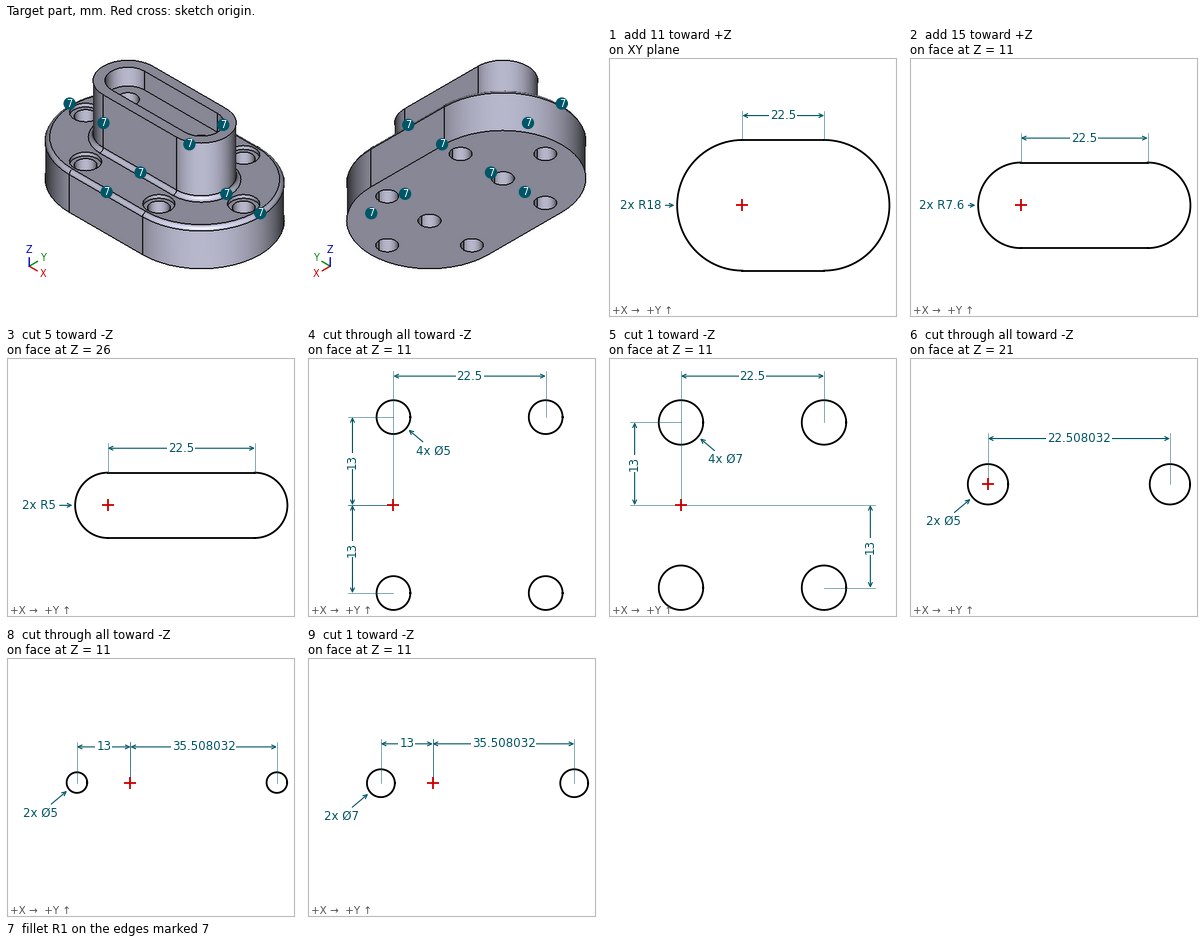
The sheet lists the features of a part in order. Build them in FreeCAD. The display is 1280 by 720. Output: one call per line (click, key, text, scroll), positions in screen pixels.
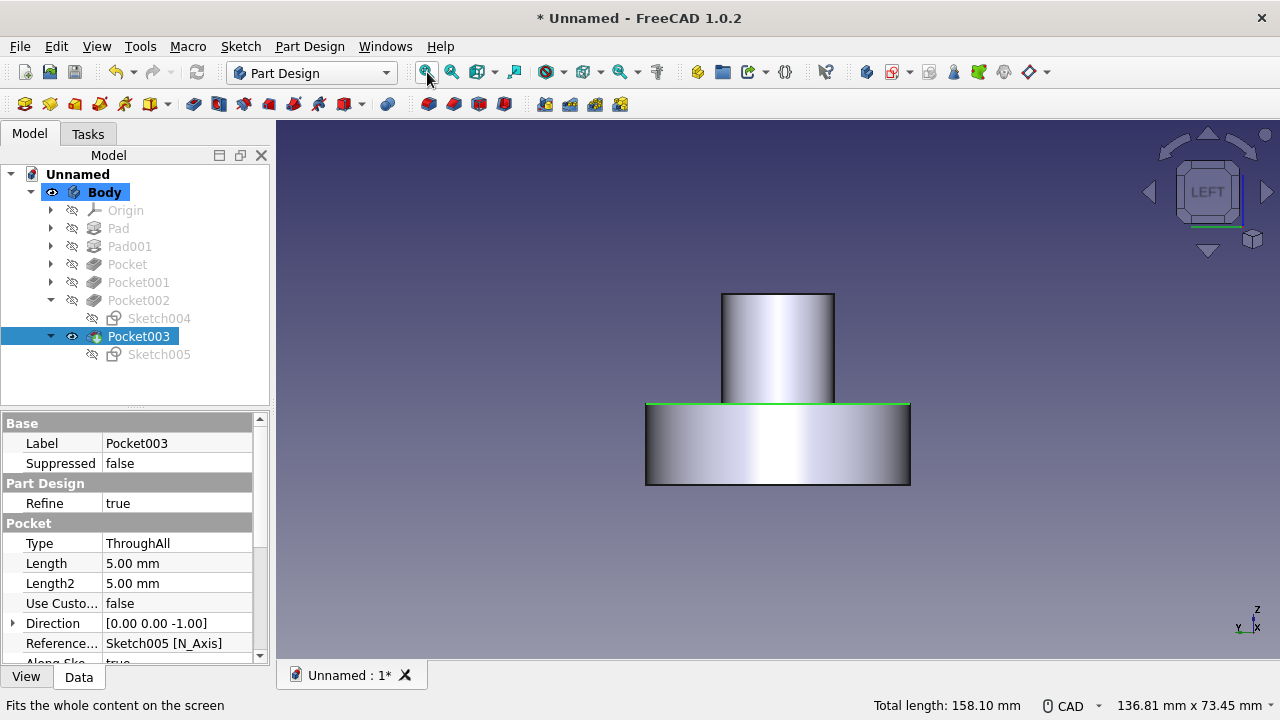
click(427, 72)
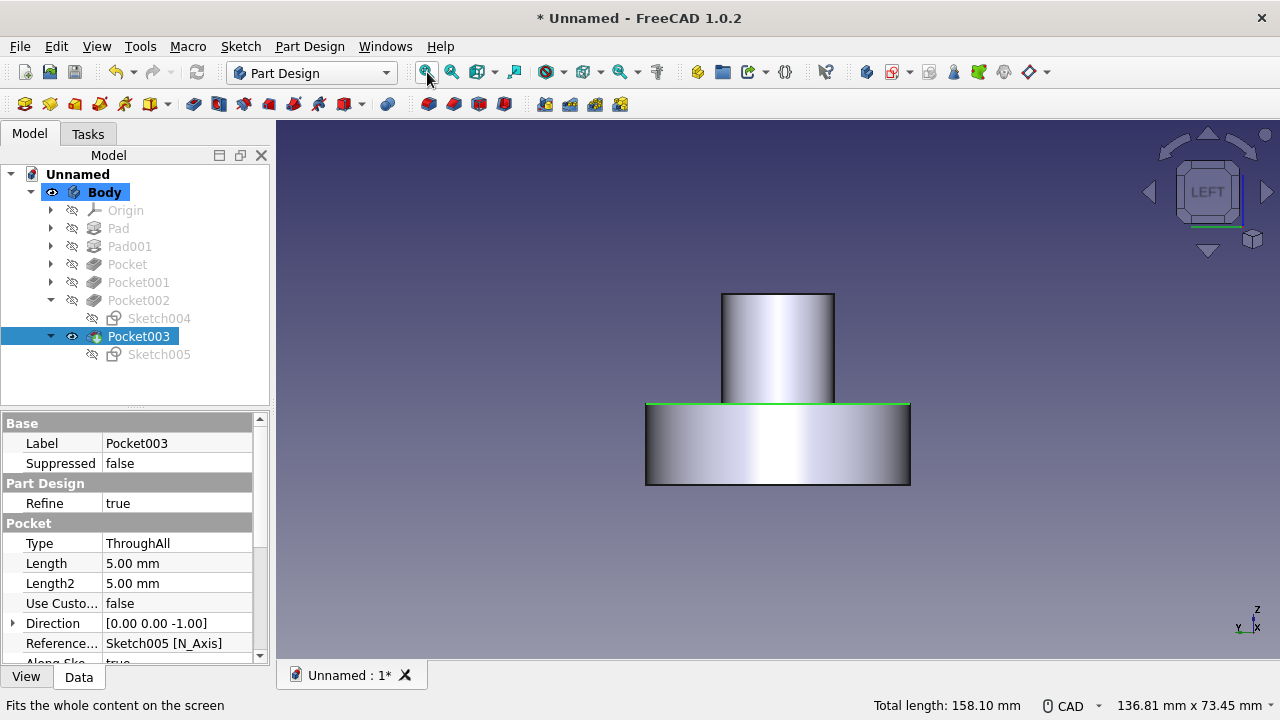
key(v)
key(3)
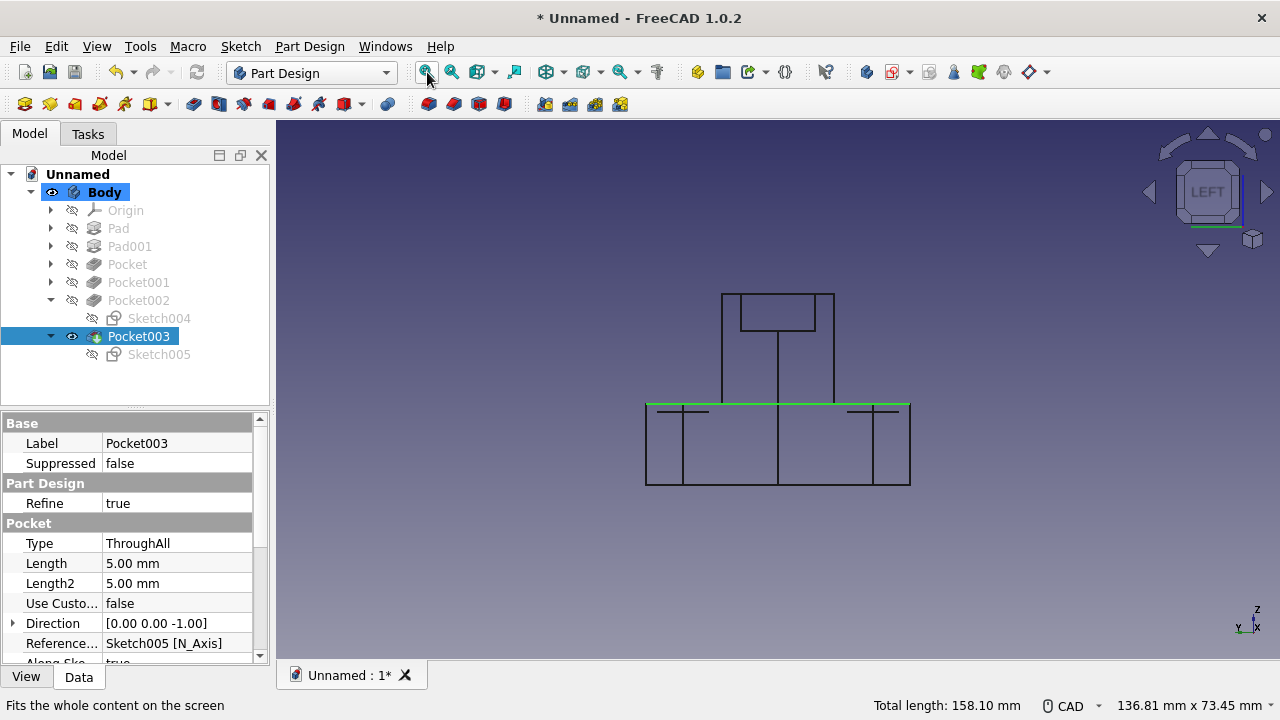
key(0)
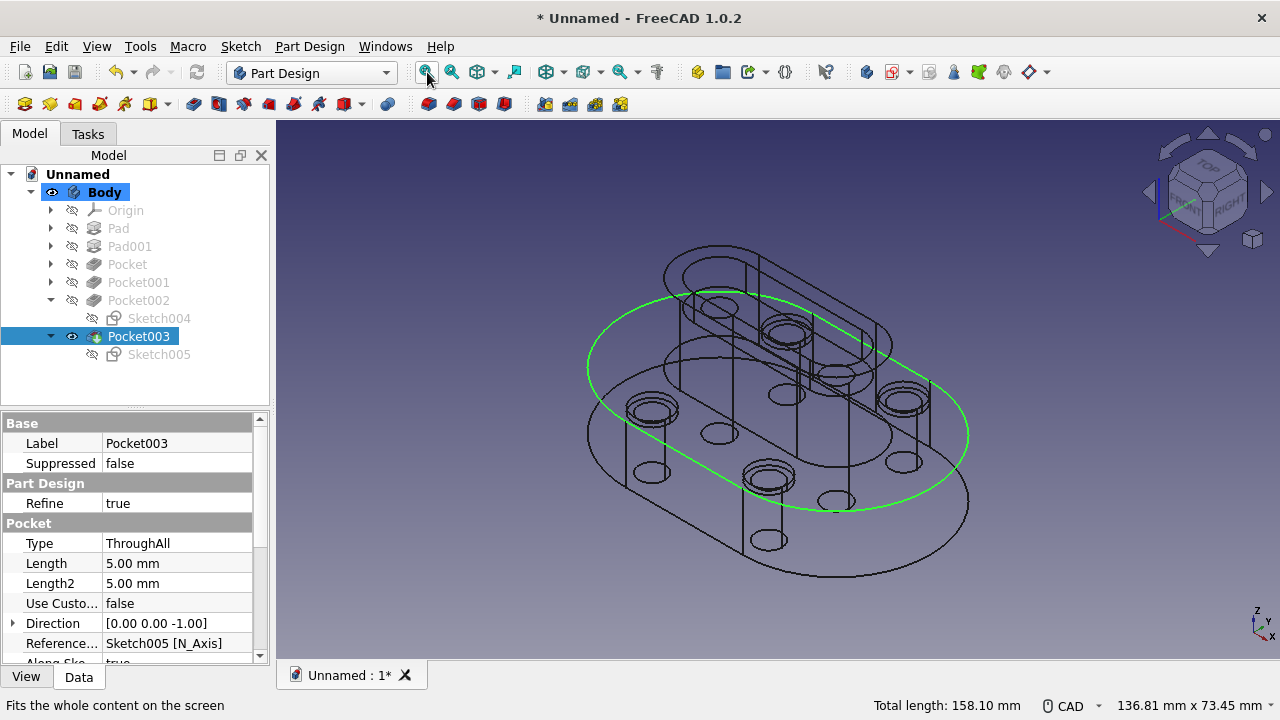
click(694, 338, ctrl)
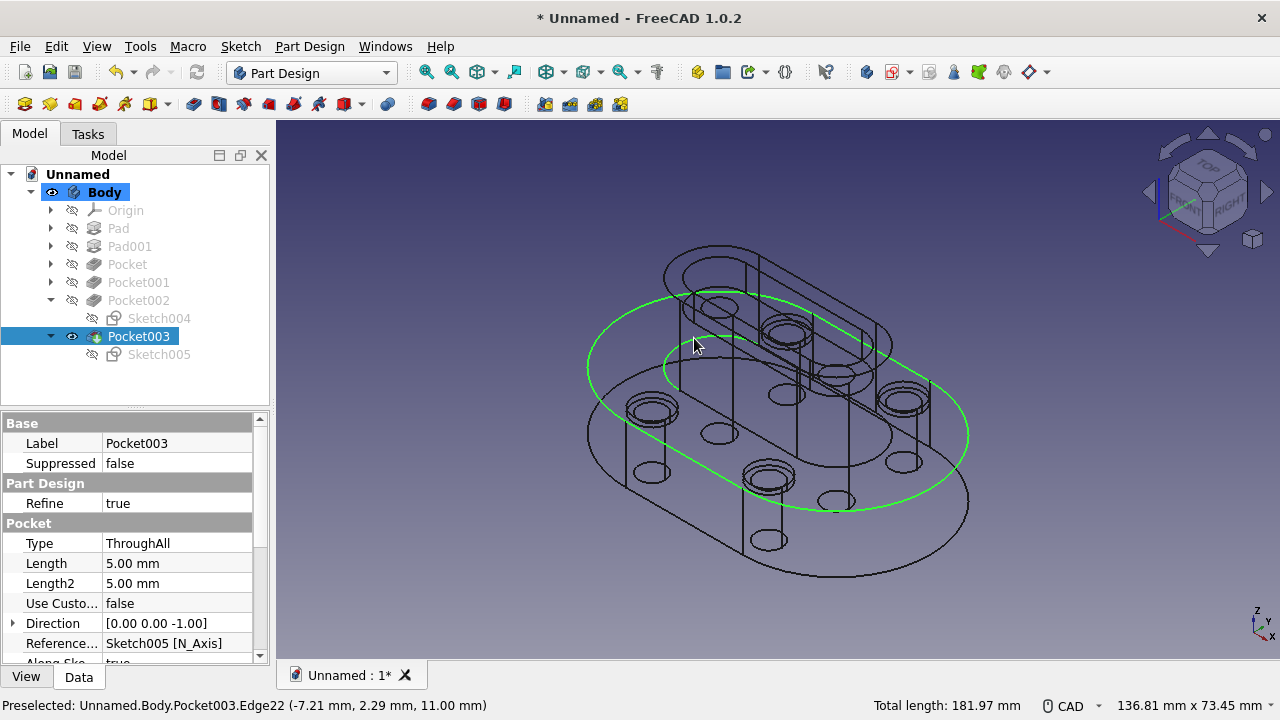
click(739, 423, ctrl)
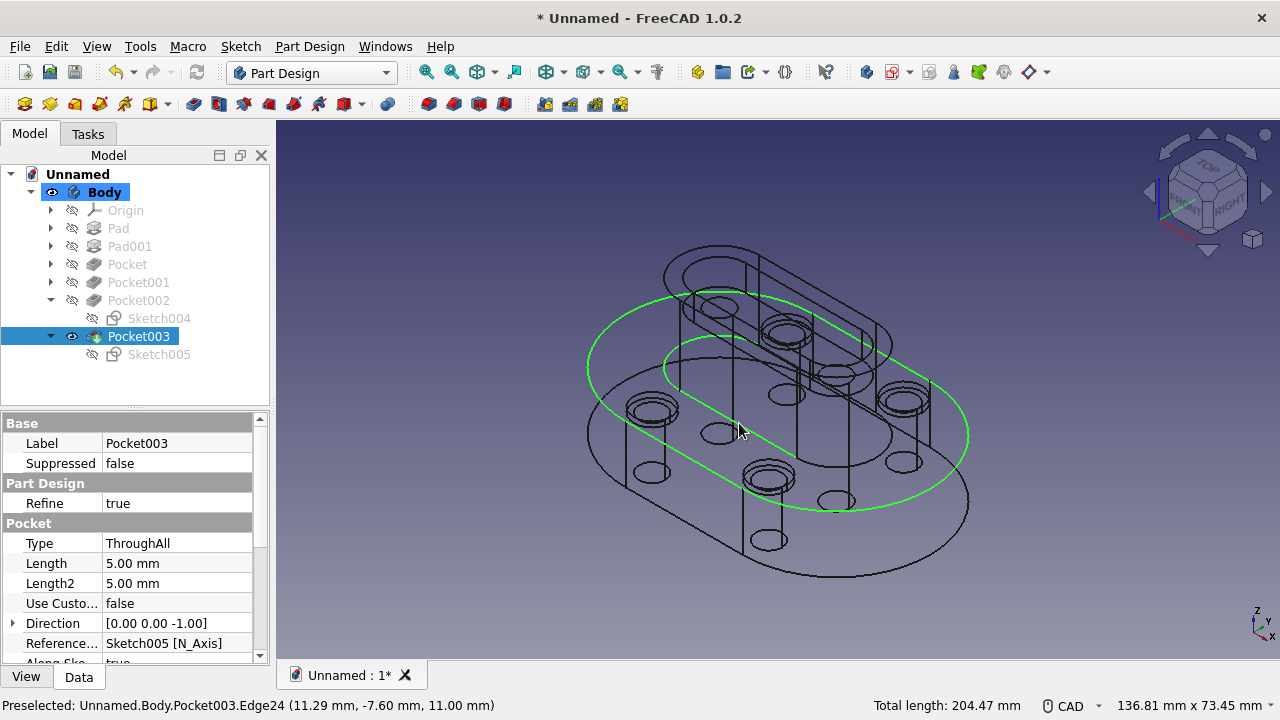
click(876, 457, ctrl)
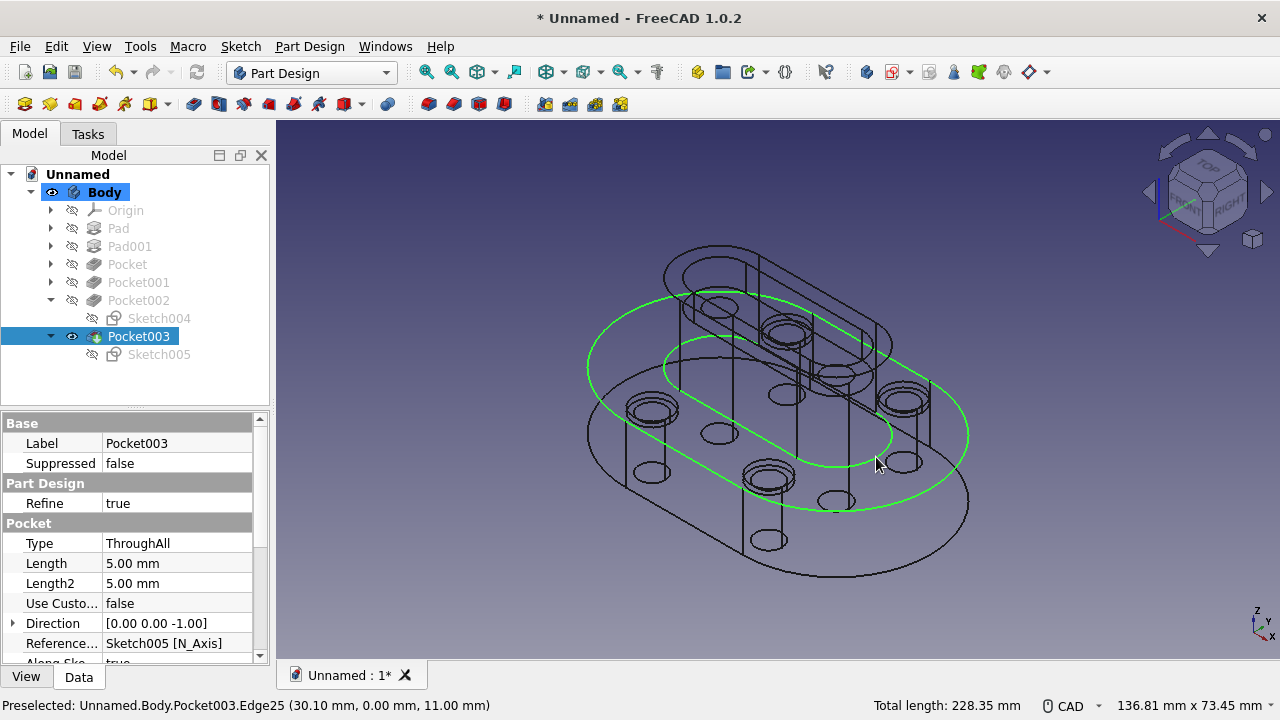
click(862, 403, ctrl)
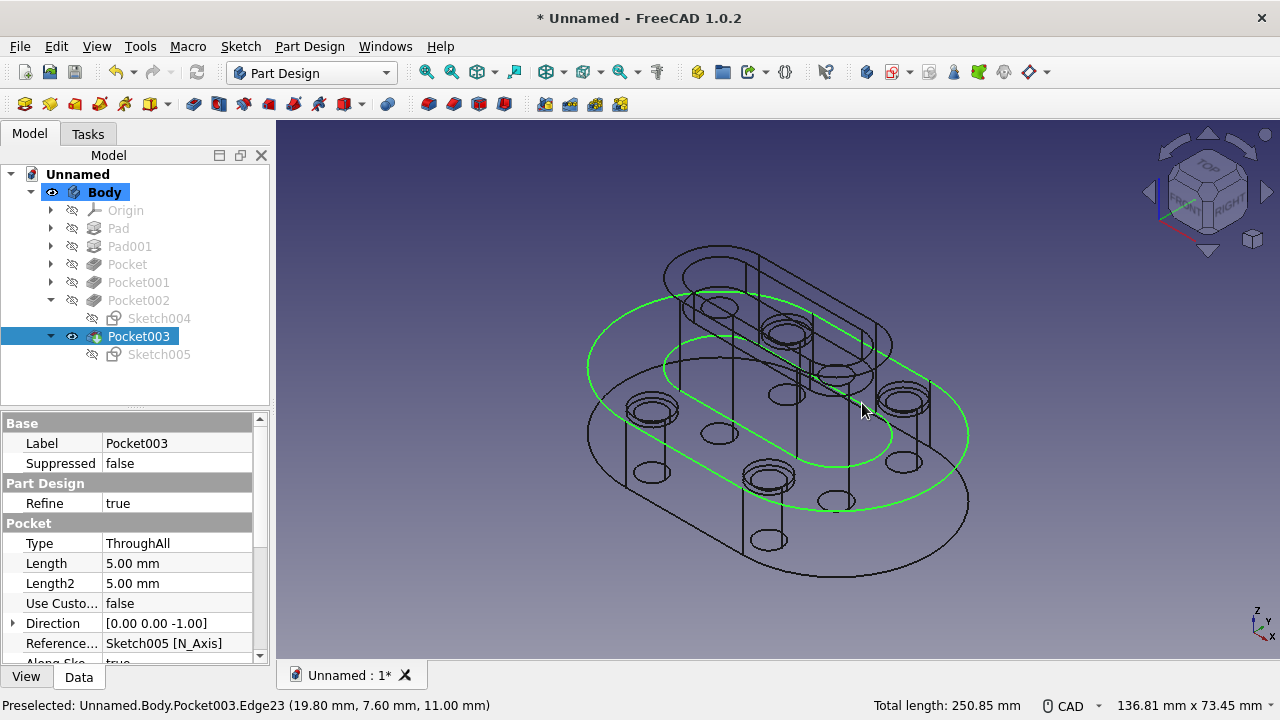
key(v)
key(1)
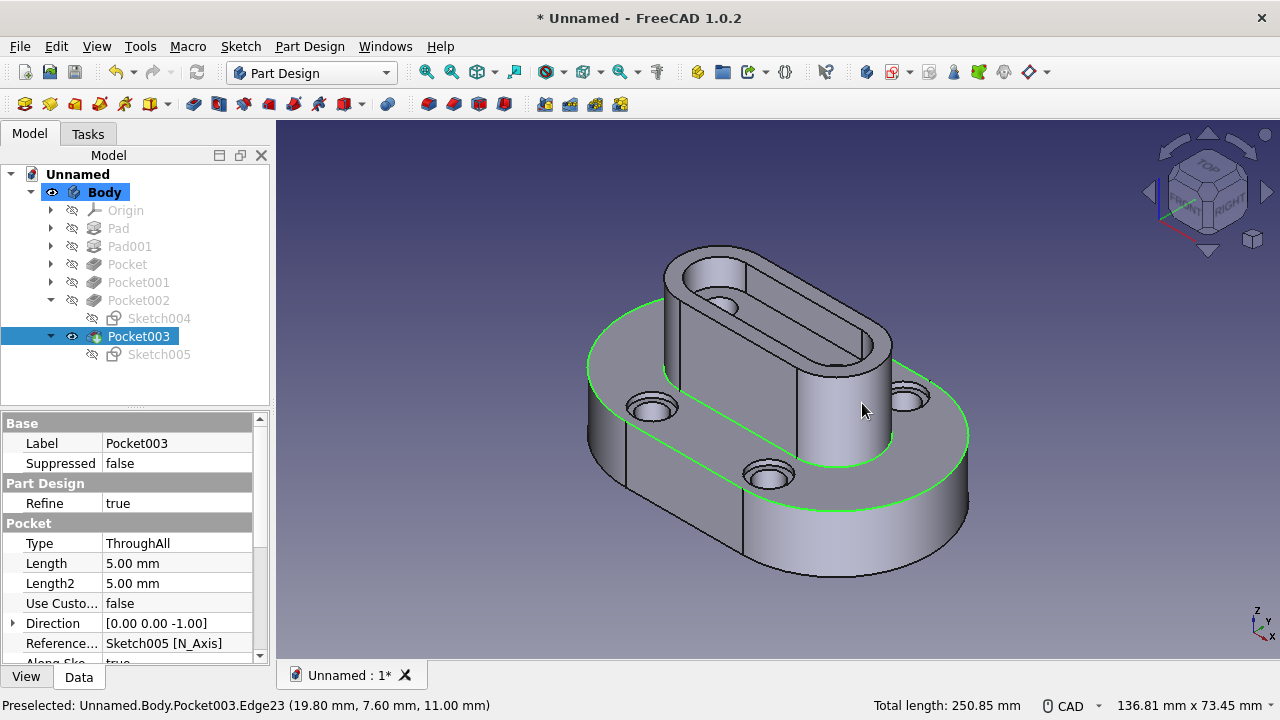
click(429, 104)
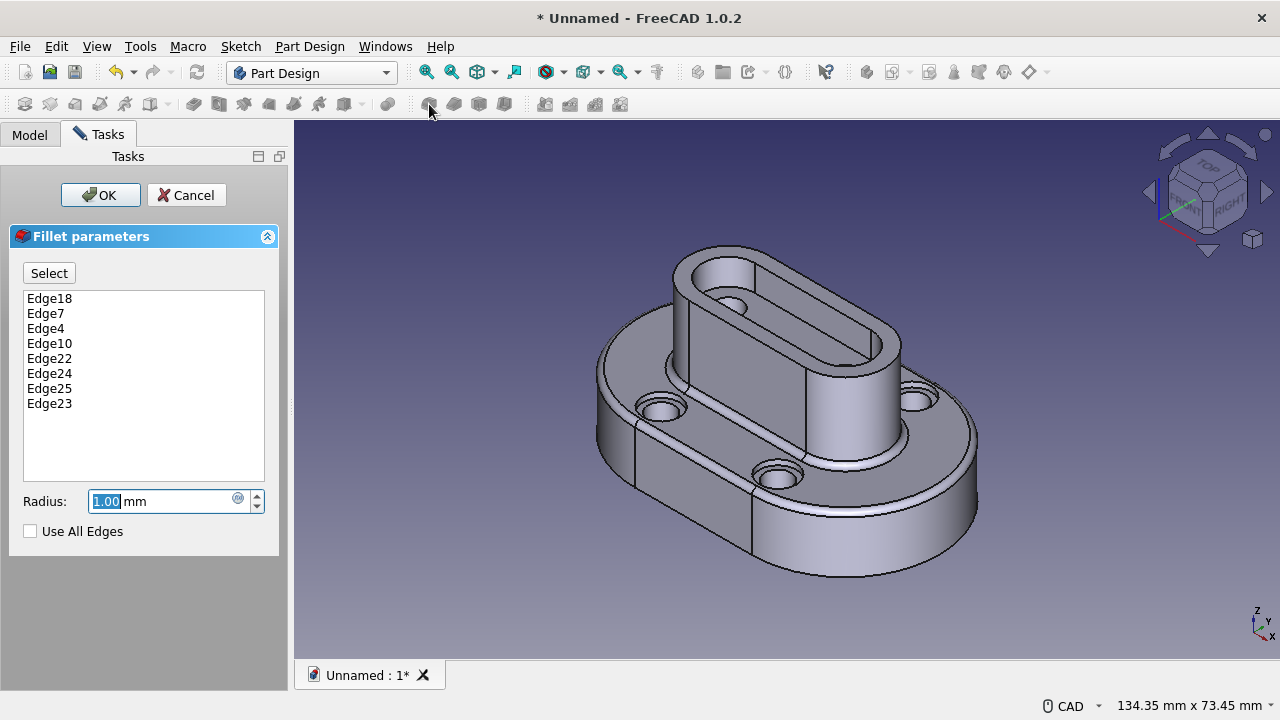
text(1)
key(Tab)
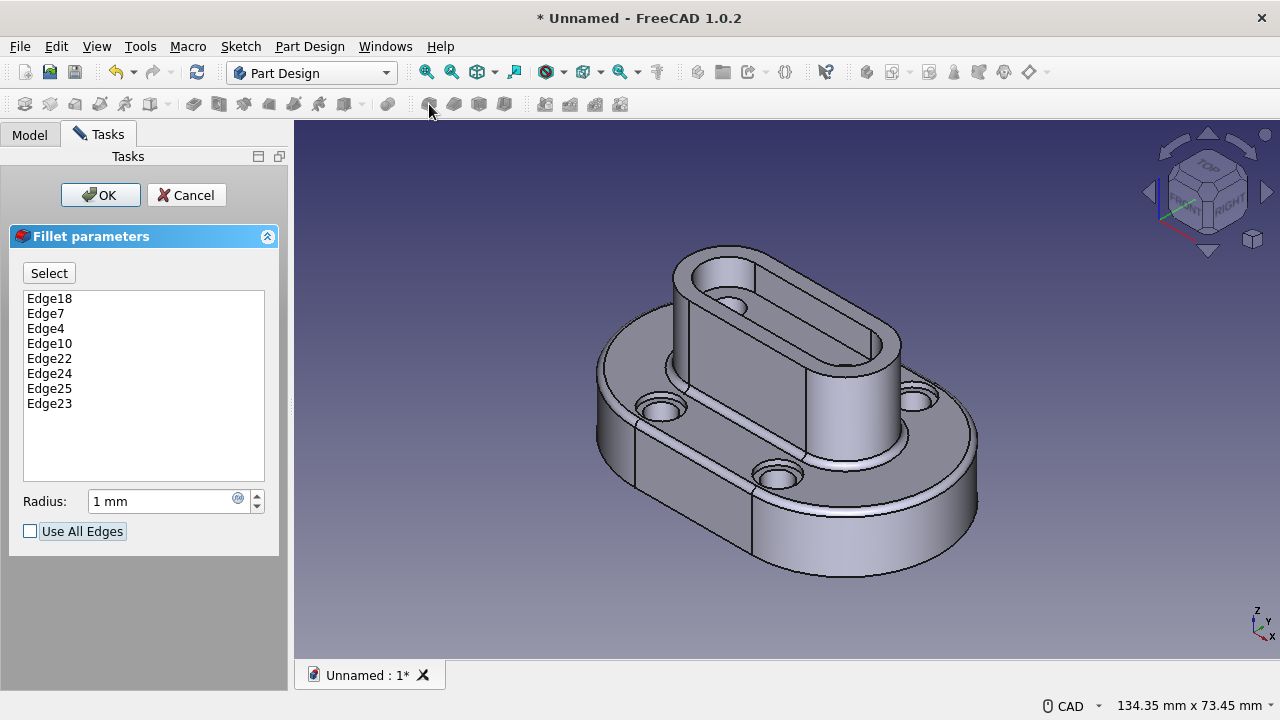
click(101, 195)